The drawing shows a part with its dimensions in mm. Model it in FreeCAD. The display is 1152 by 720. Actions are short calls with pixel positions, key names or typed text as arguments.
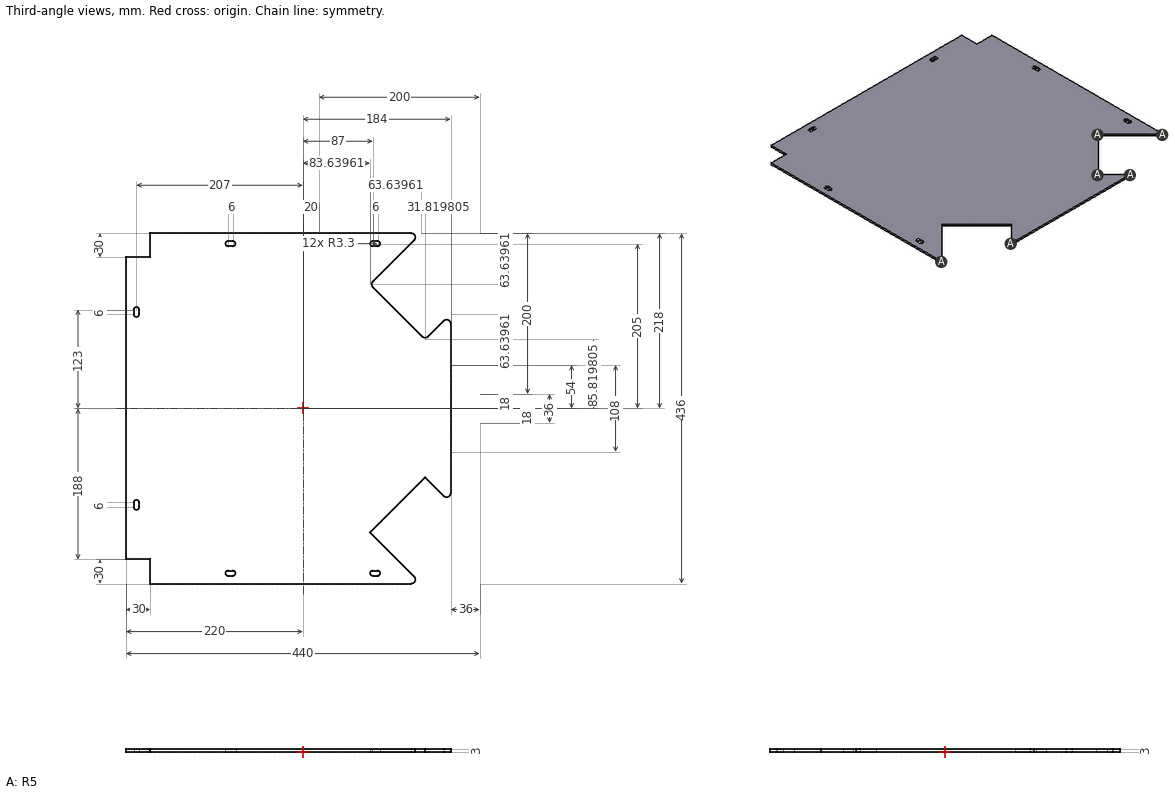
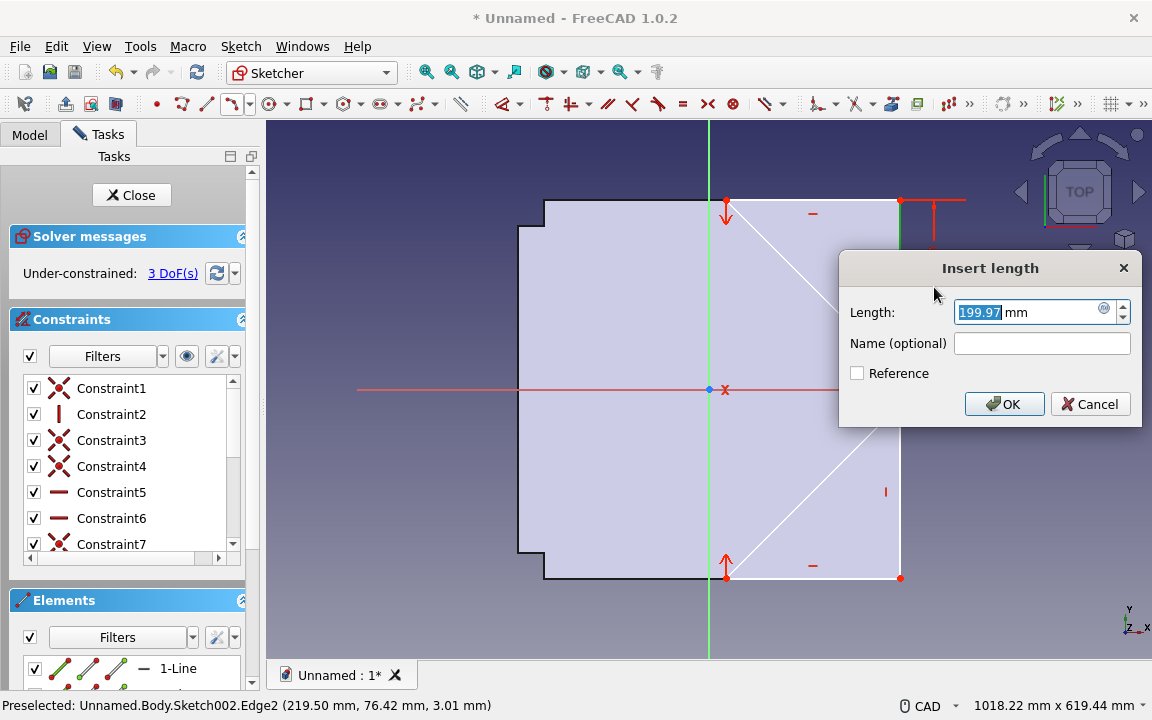
text(200)
key(Return)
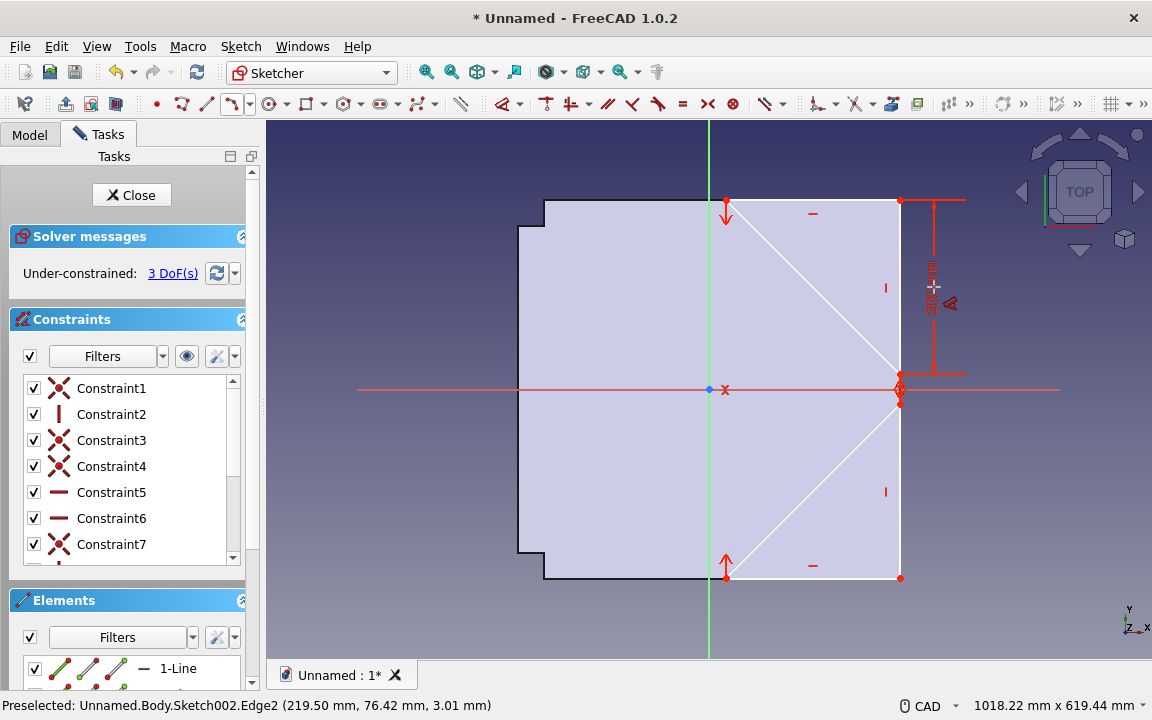
click(848, 200)
click(813, 166)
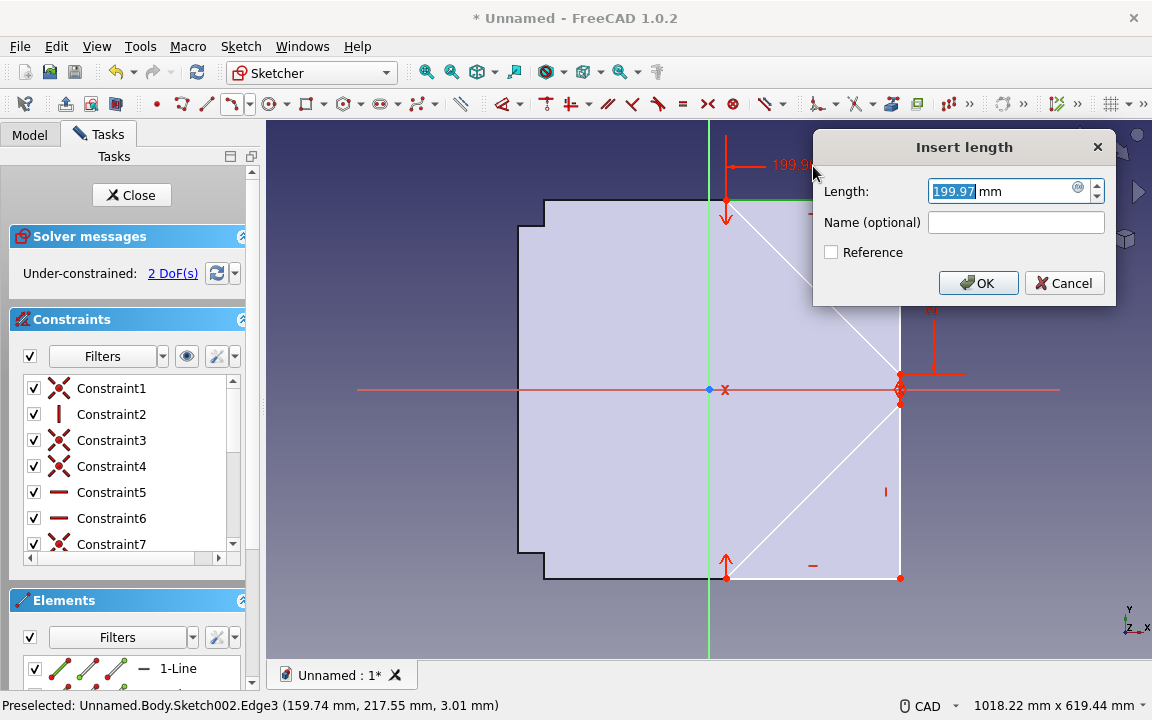
text(200)
key(Return)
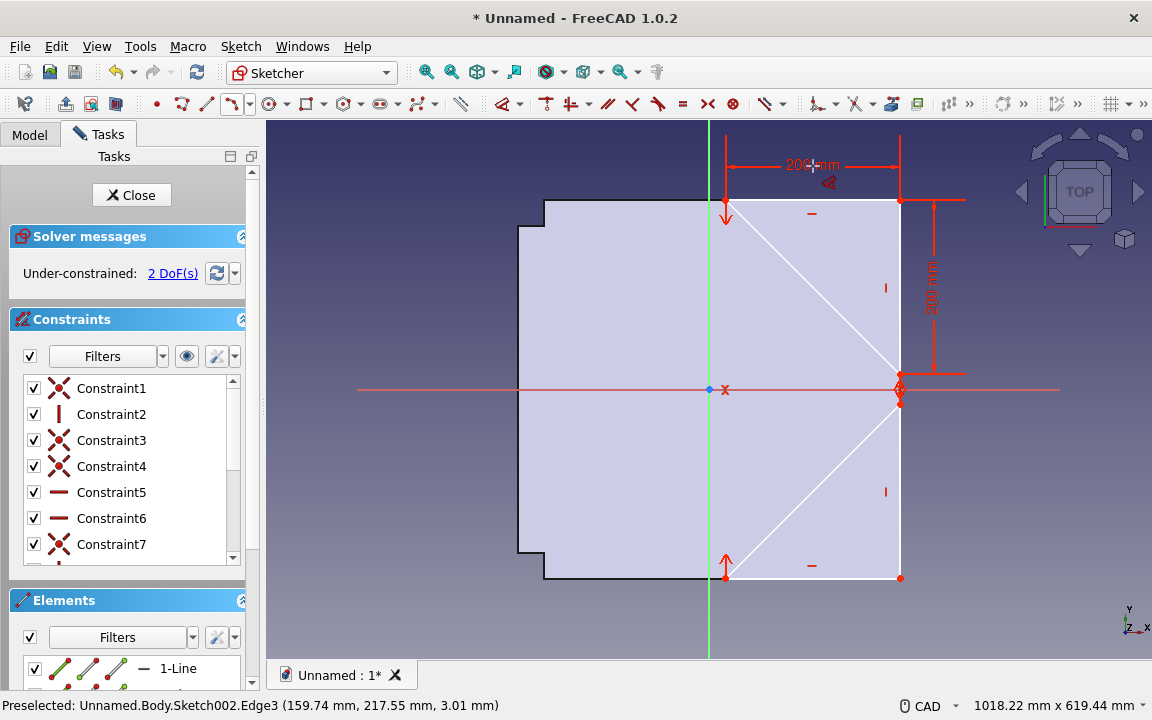
scroll(726, 200, up, 5)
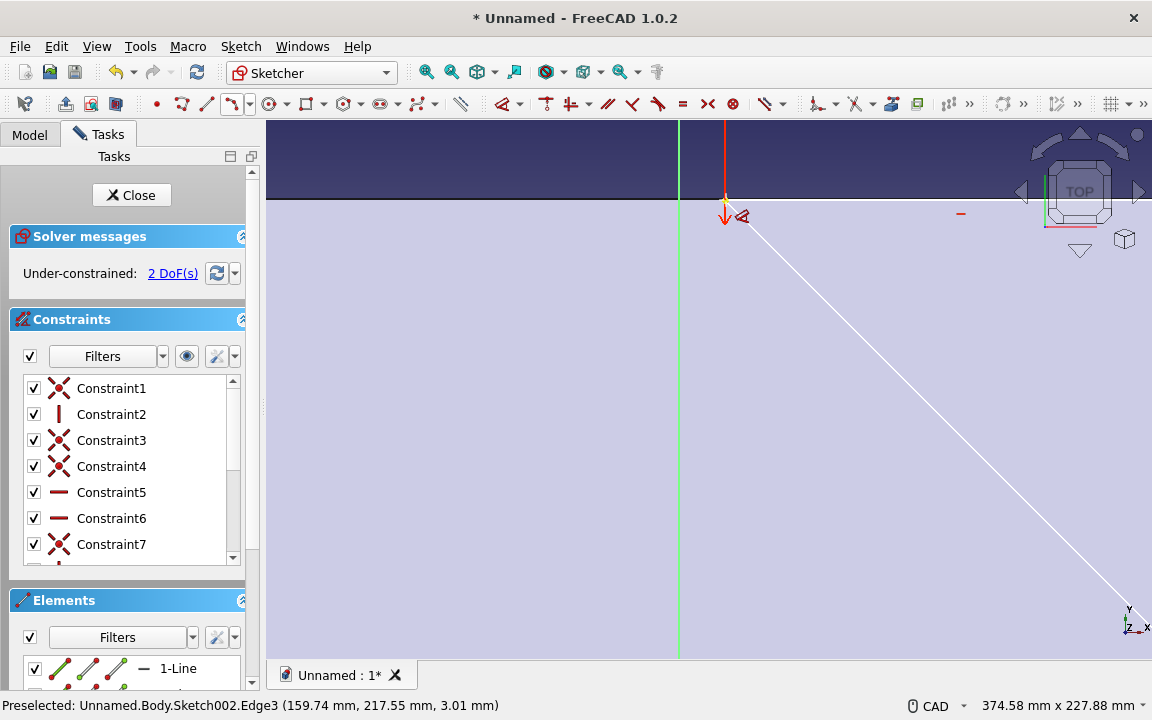
click(725, 200)
click(702, 166)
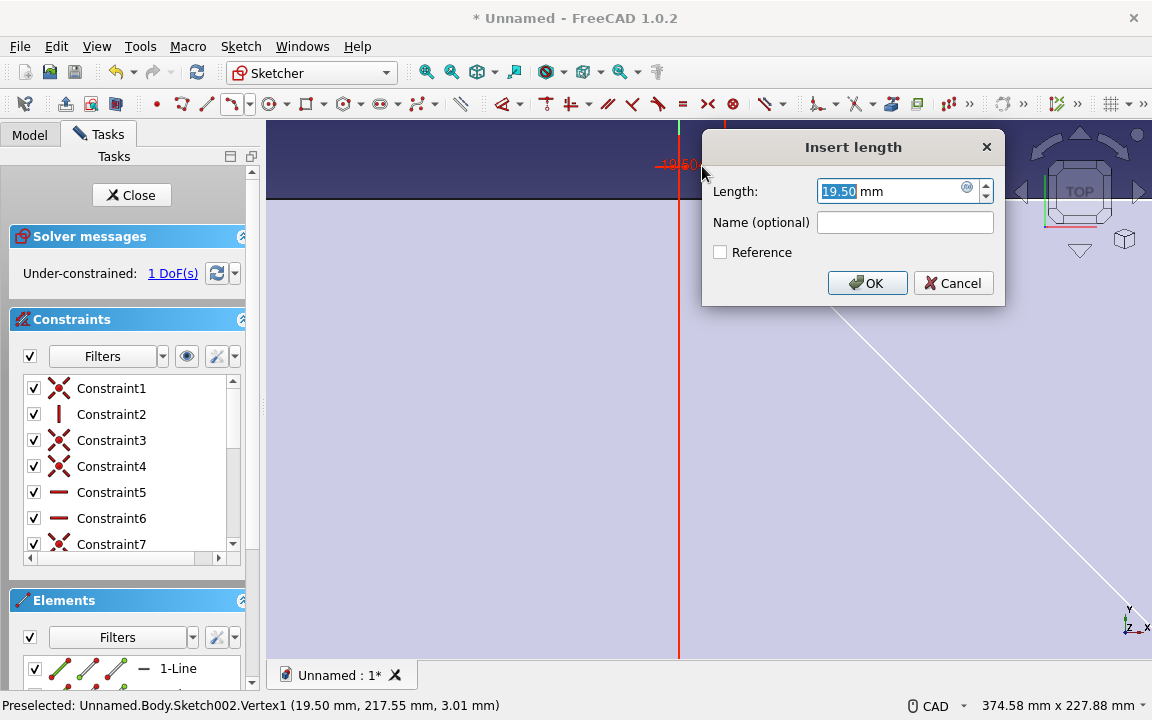
text(20)
key(Return)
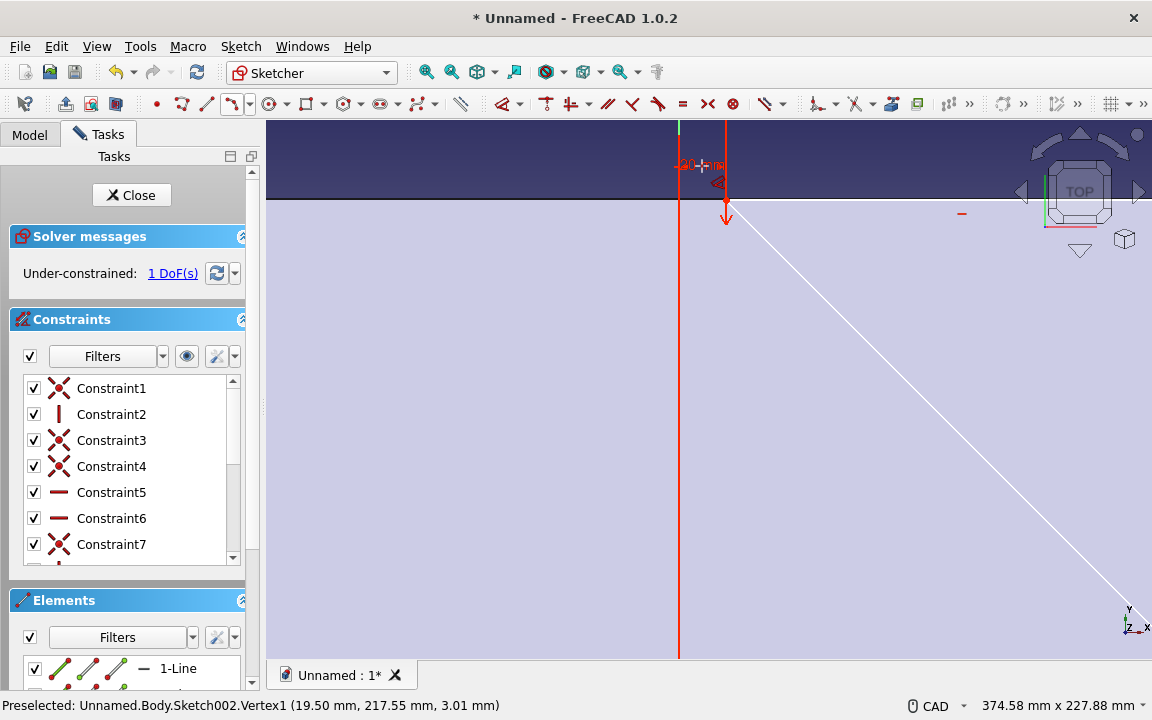
scroll(512, 249, down, 6)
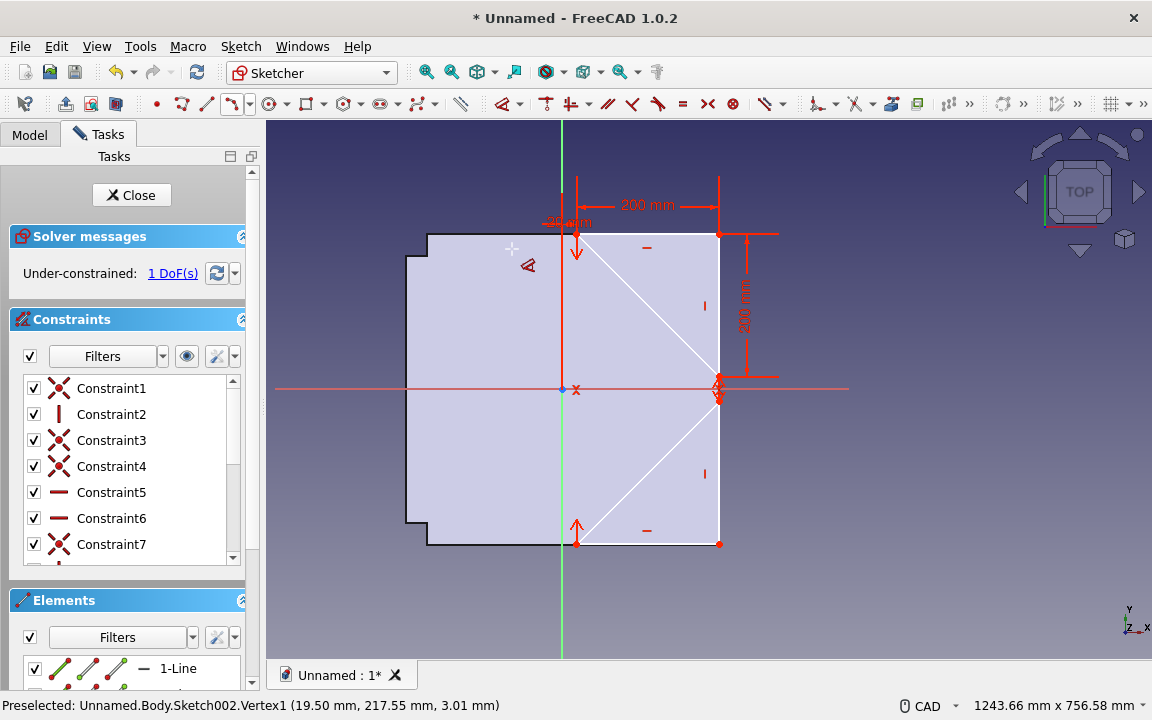
scroll(719, 377, up, 6)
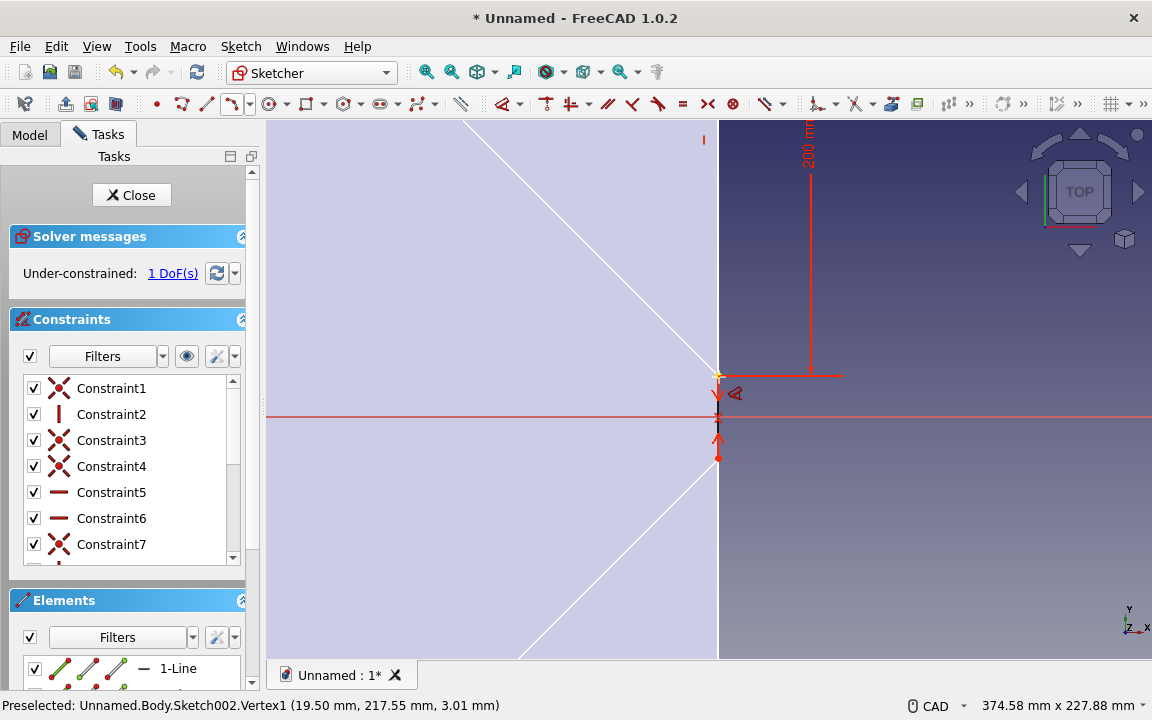
click(718, 376)
click(752, 397)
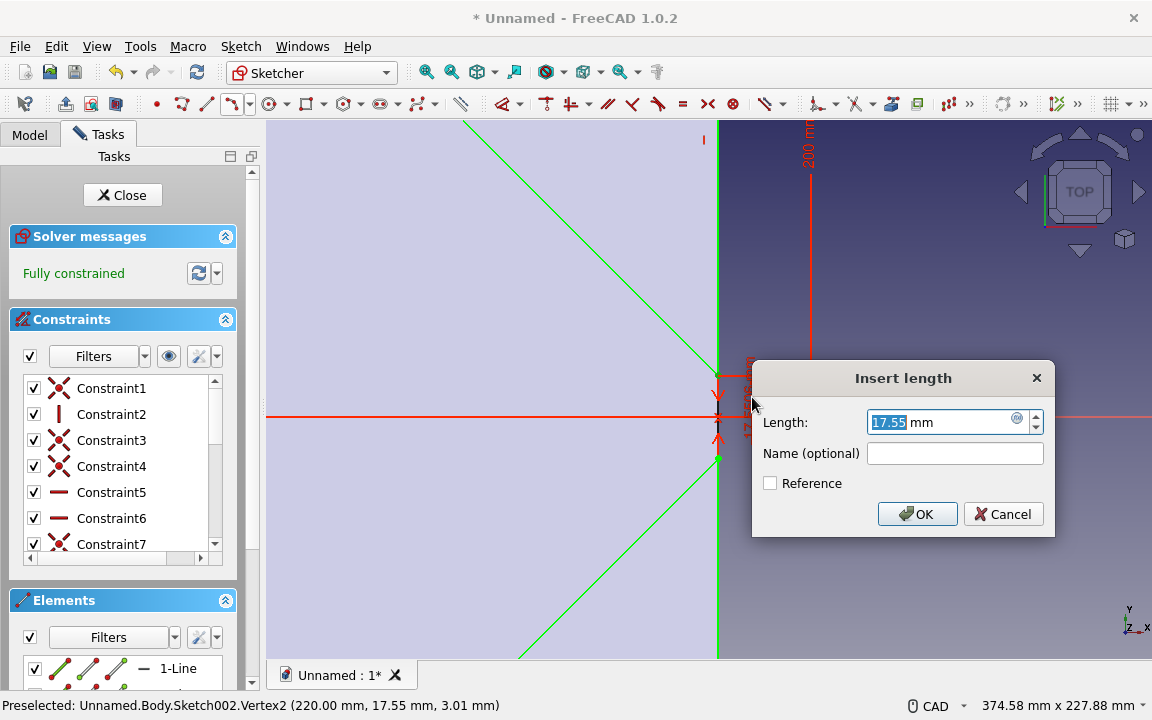
text(18)
key(Return)
key(Escape)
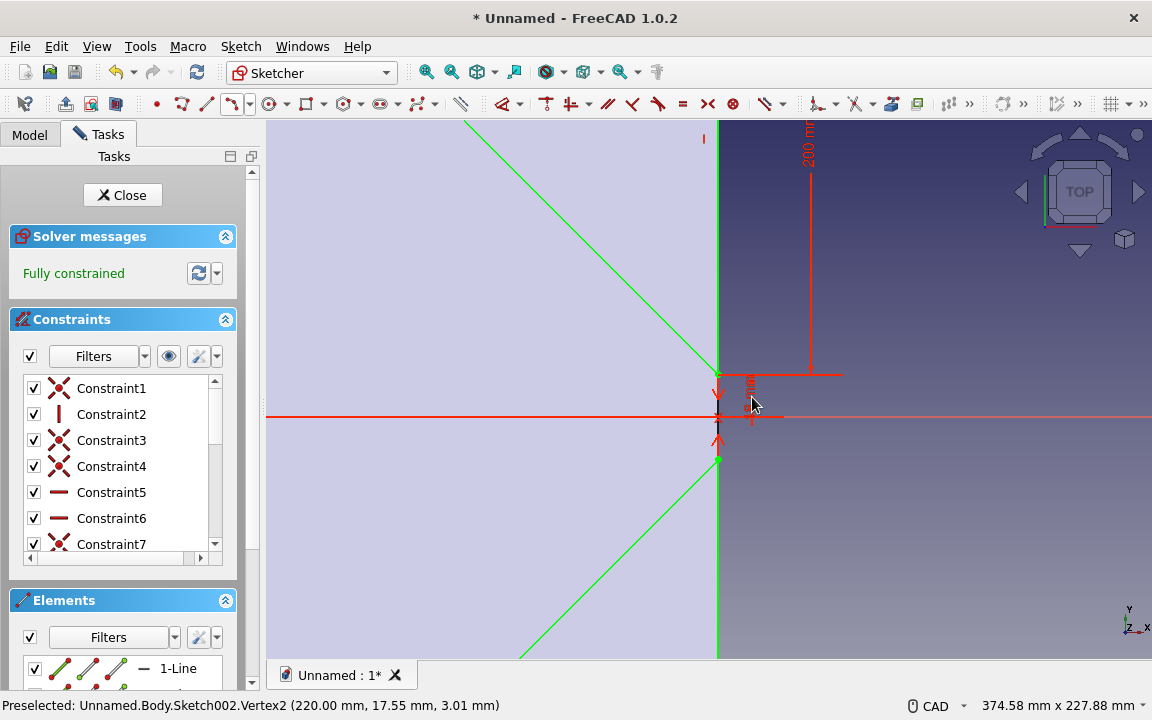
click(123, 195)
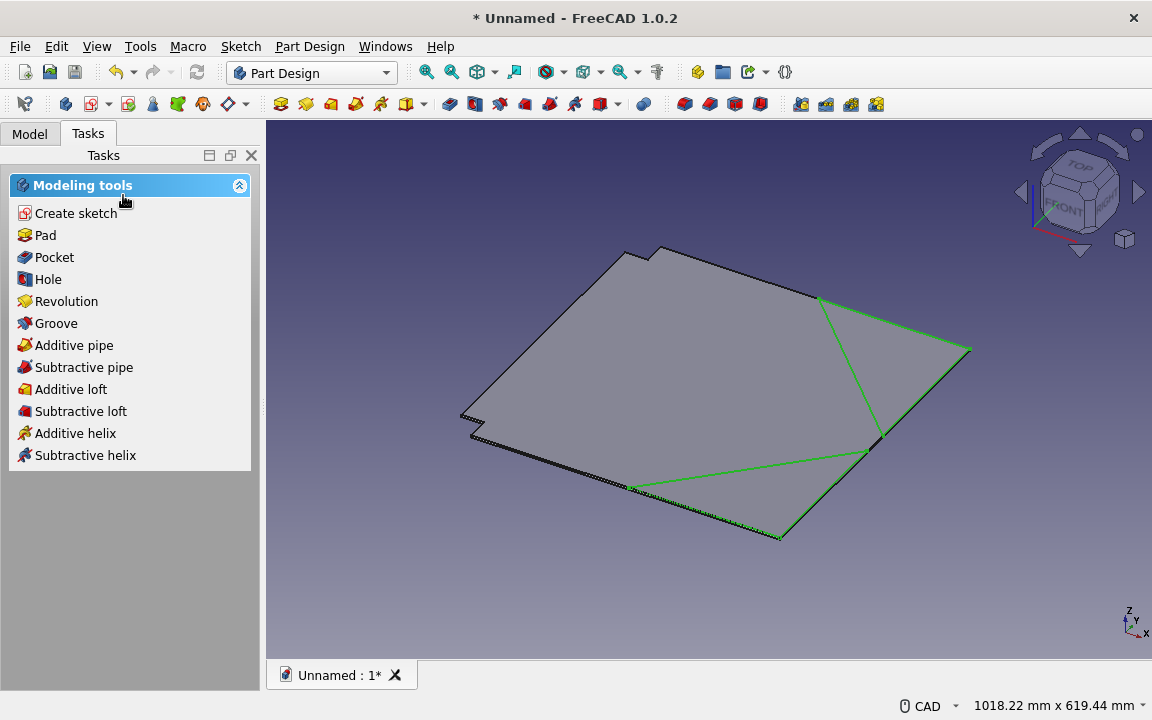
click(450, 104)